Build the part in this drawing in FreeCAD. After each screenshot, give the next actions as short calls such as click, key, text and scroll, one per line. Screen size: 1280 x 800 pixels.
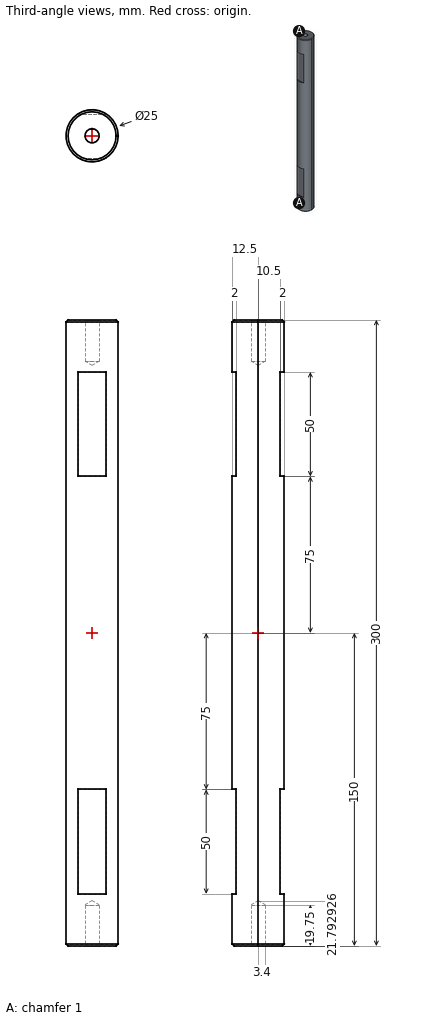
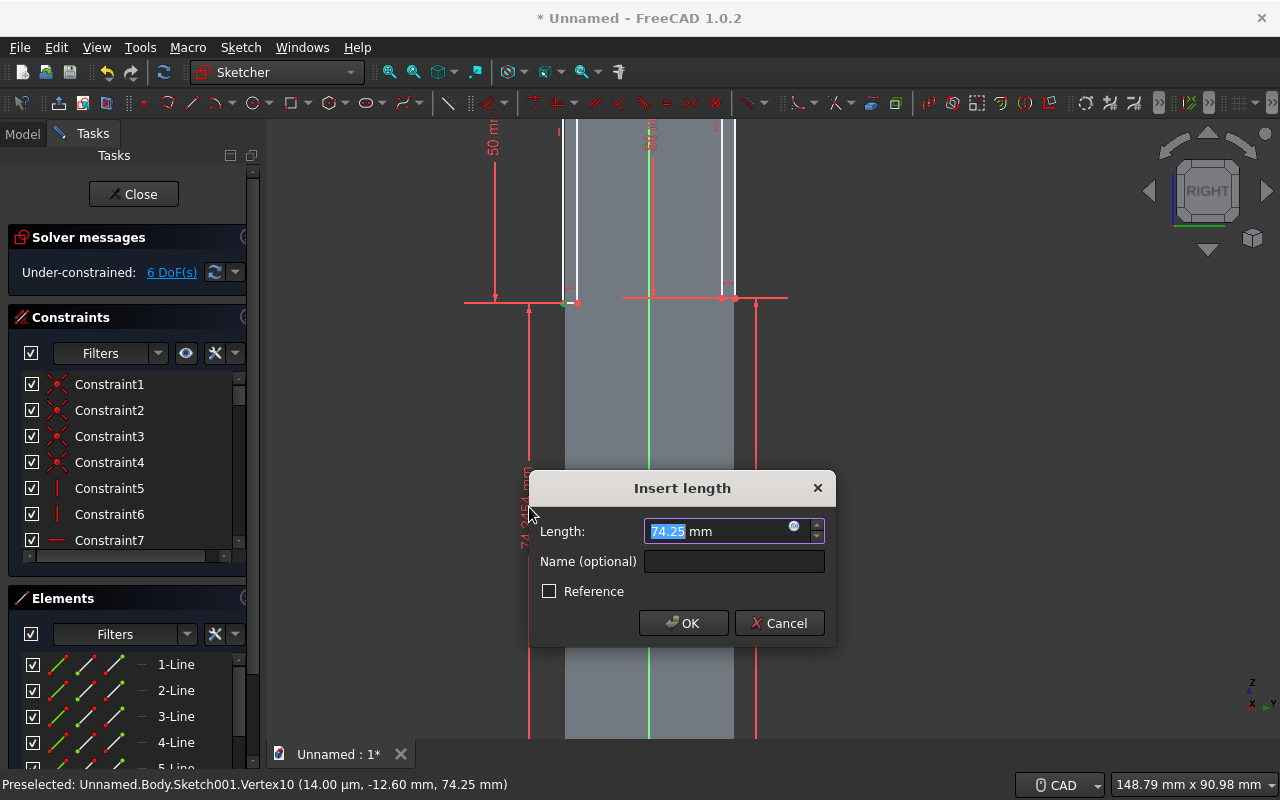
text(75)
key(Return)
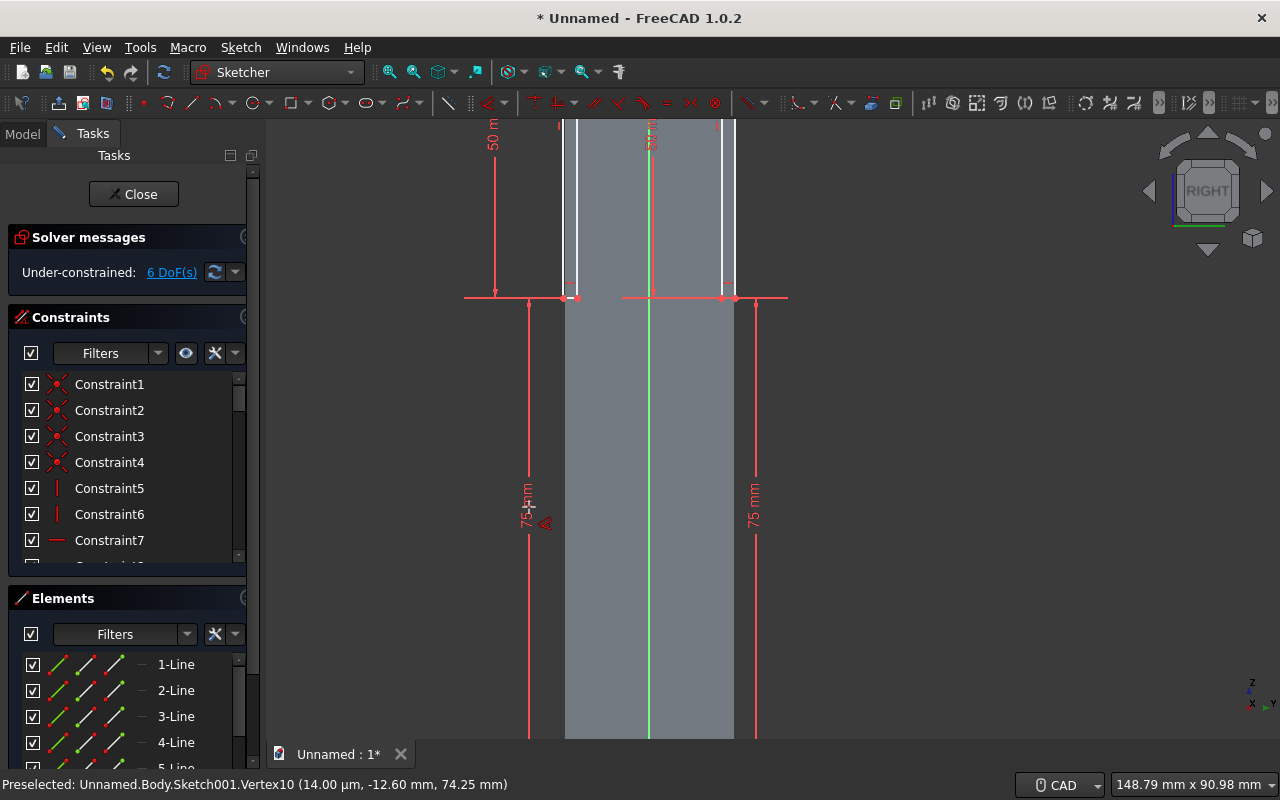
scroll(723, 305, down, 7)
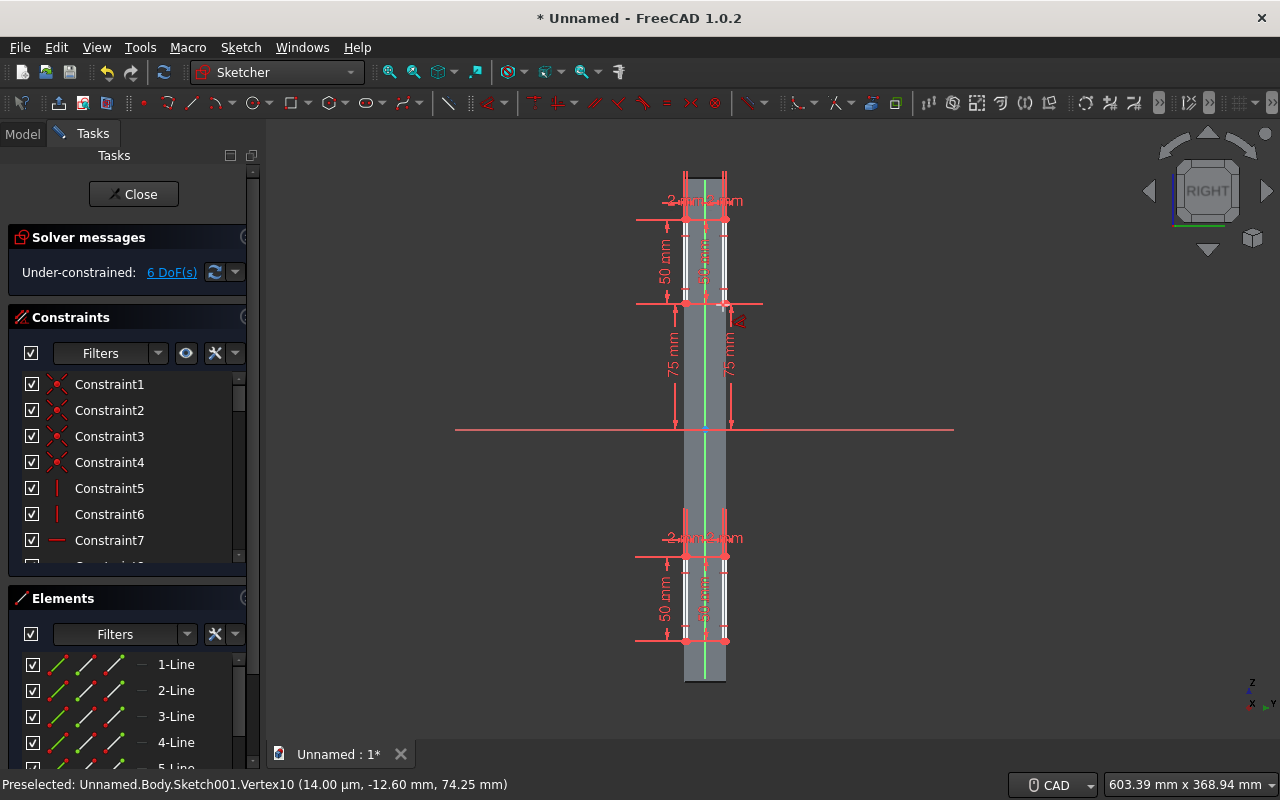
scroll(684, 557, up, 7)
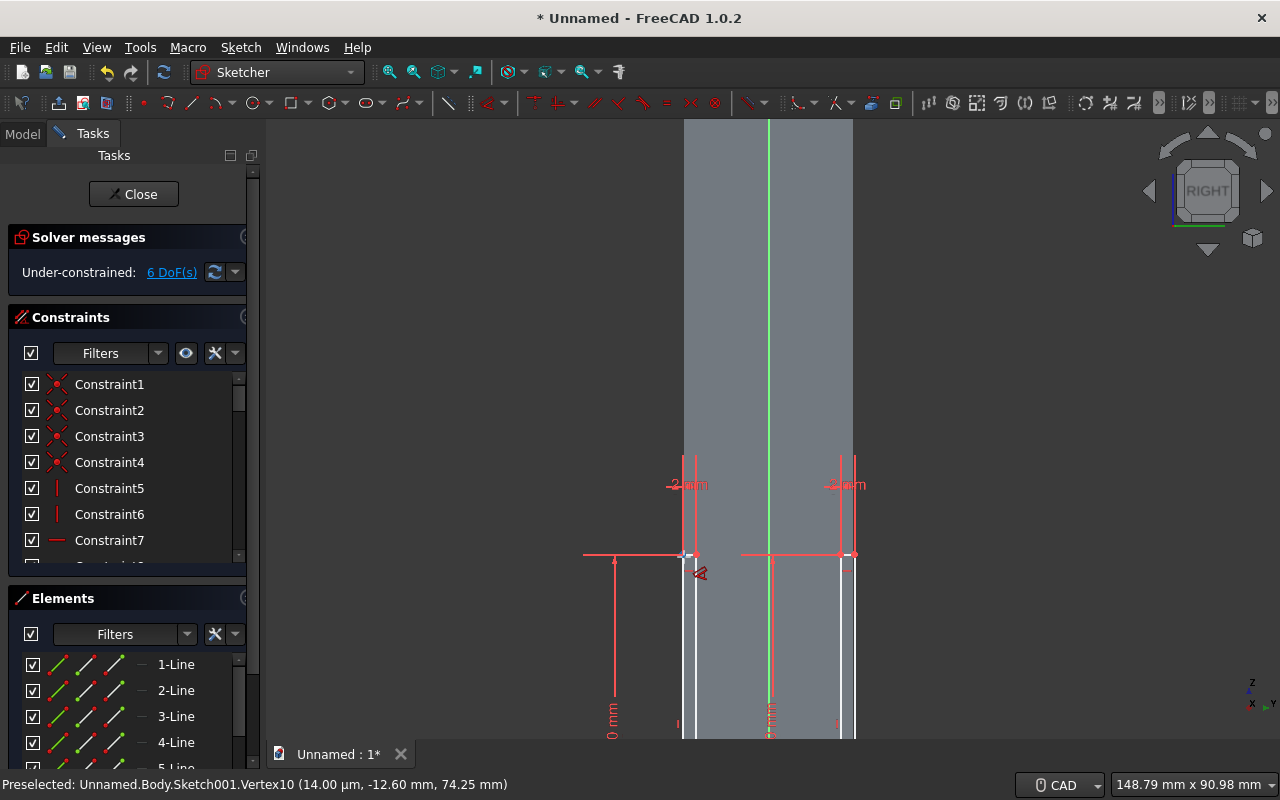
click(683, 555)
click(649, 351)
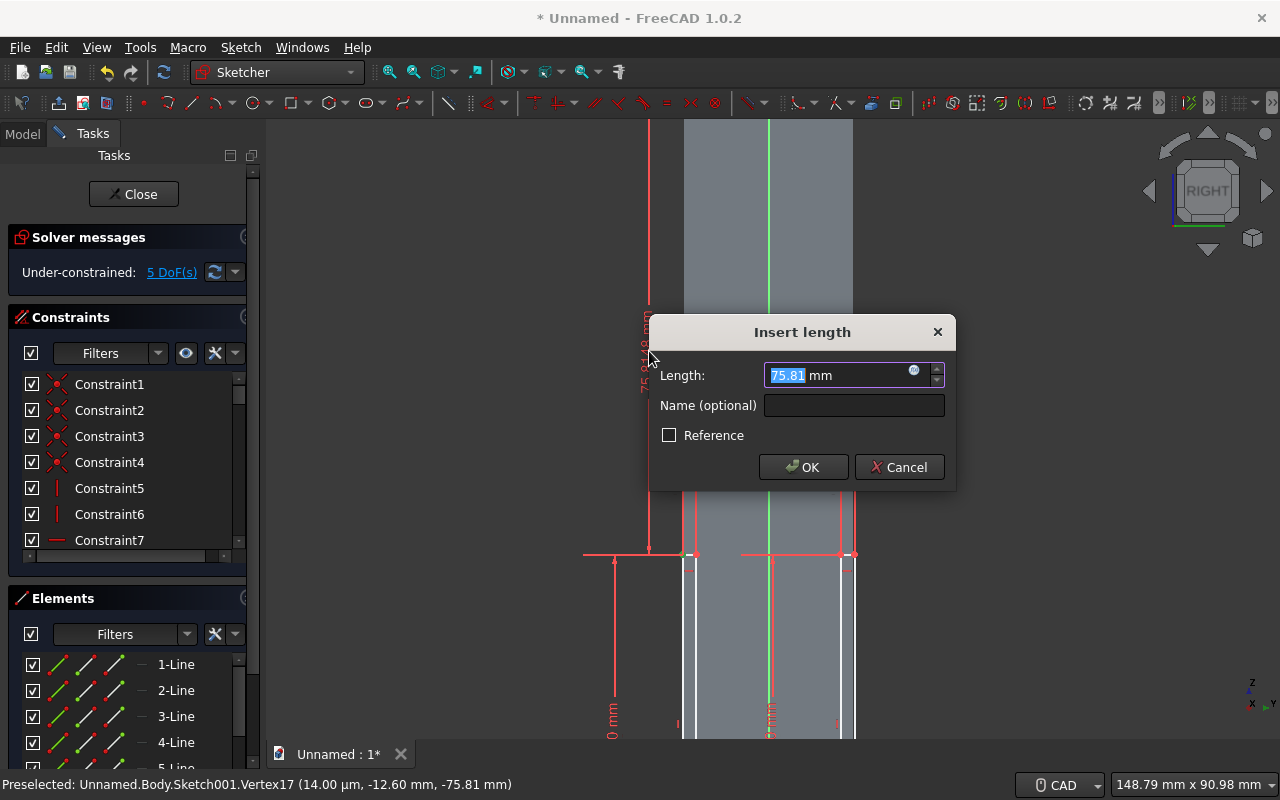
text(75)
key(Return)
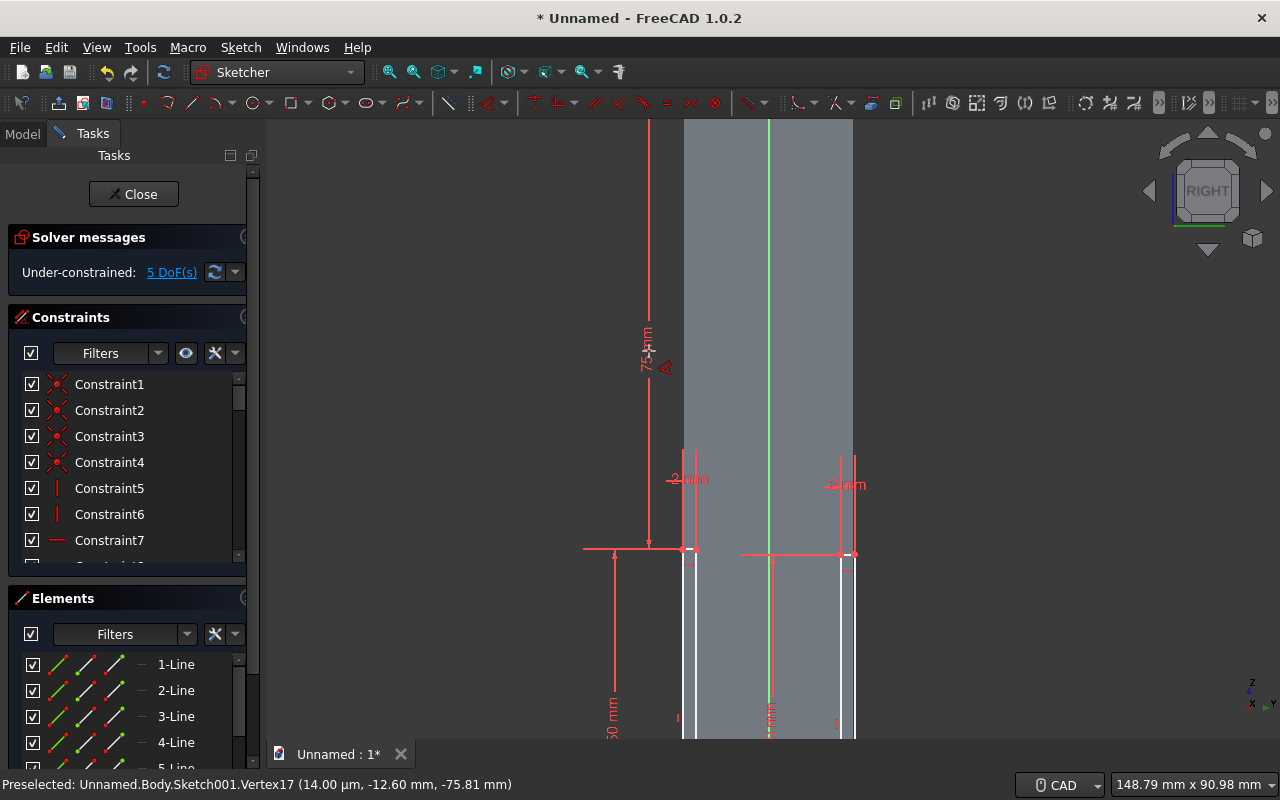
click(841, 555)
click(875, 351)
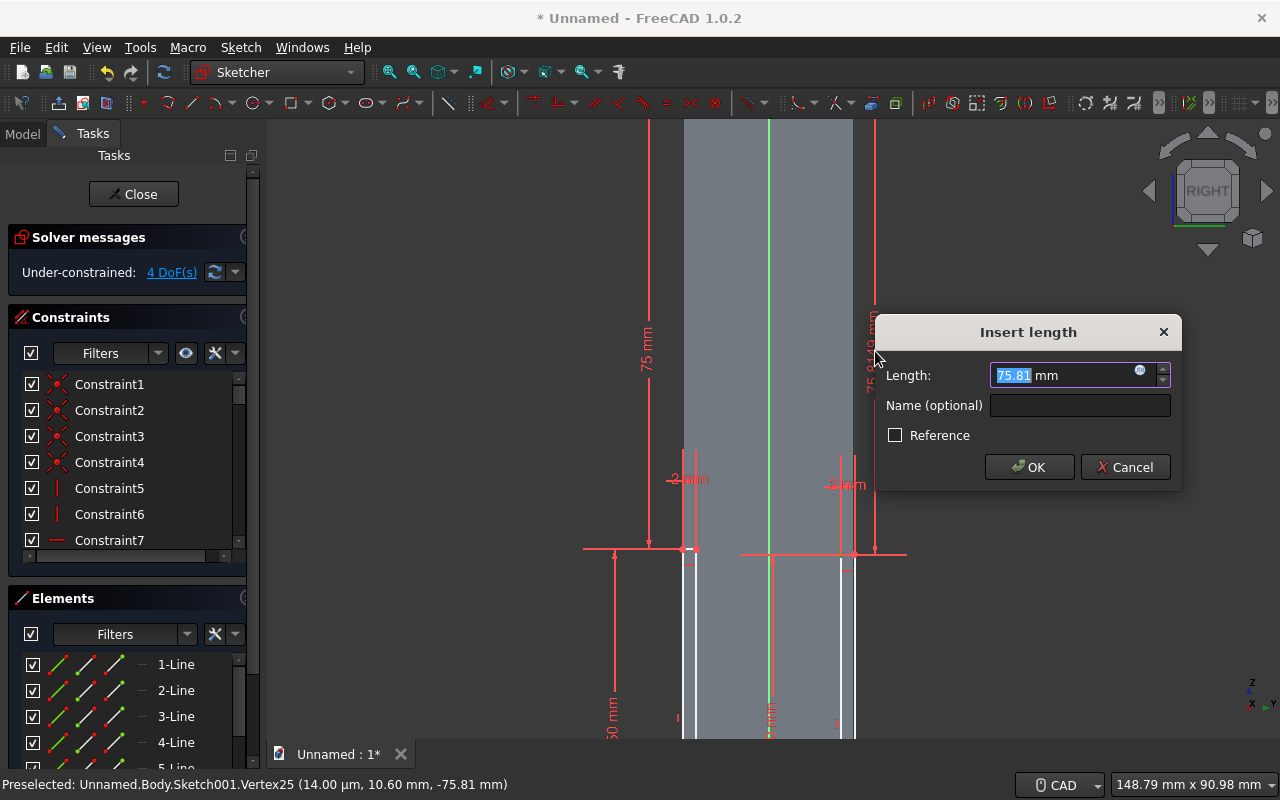
text(75)
key(Return)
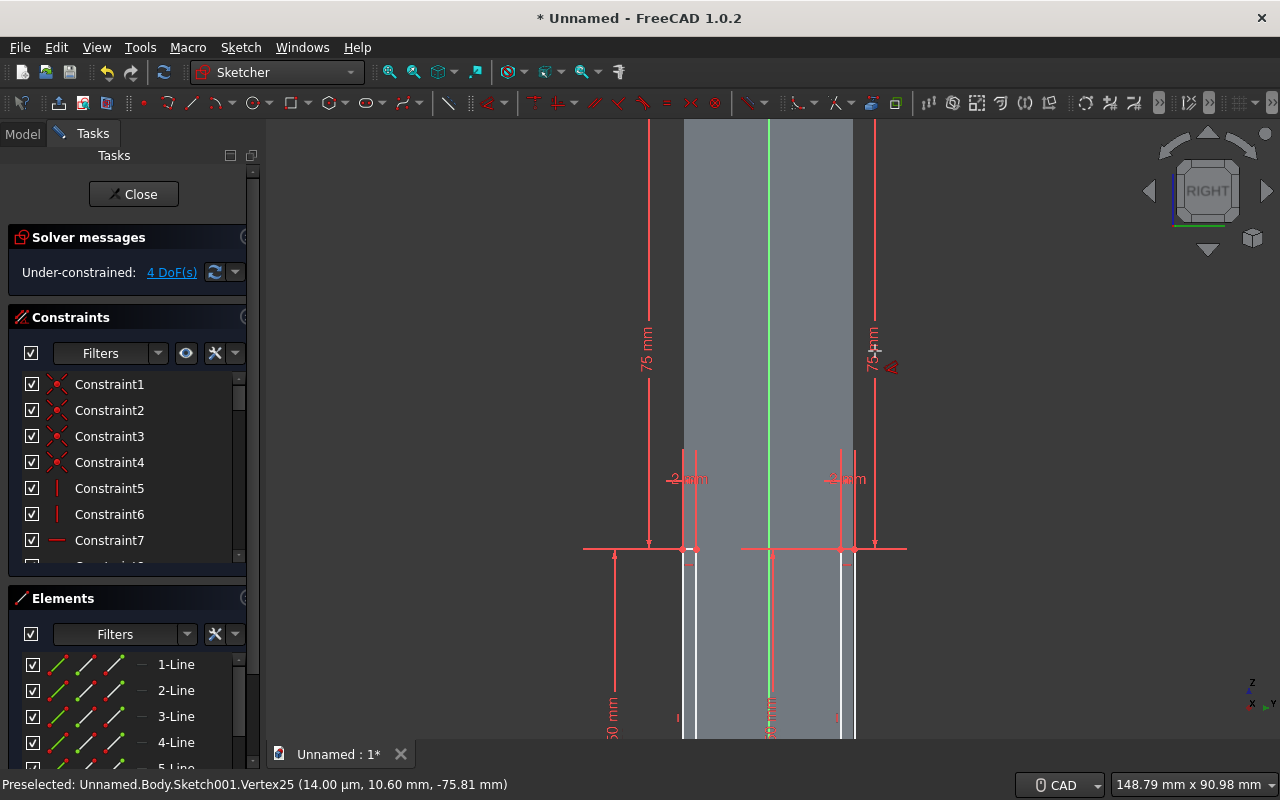
scroll(684, 557, down, 7)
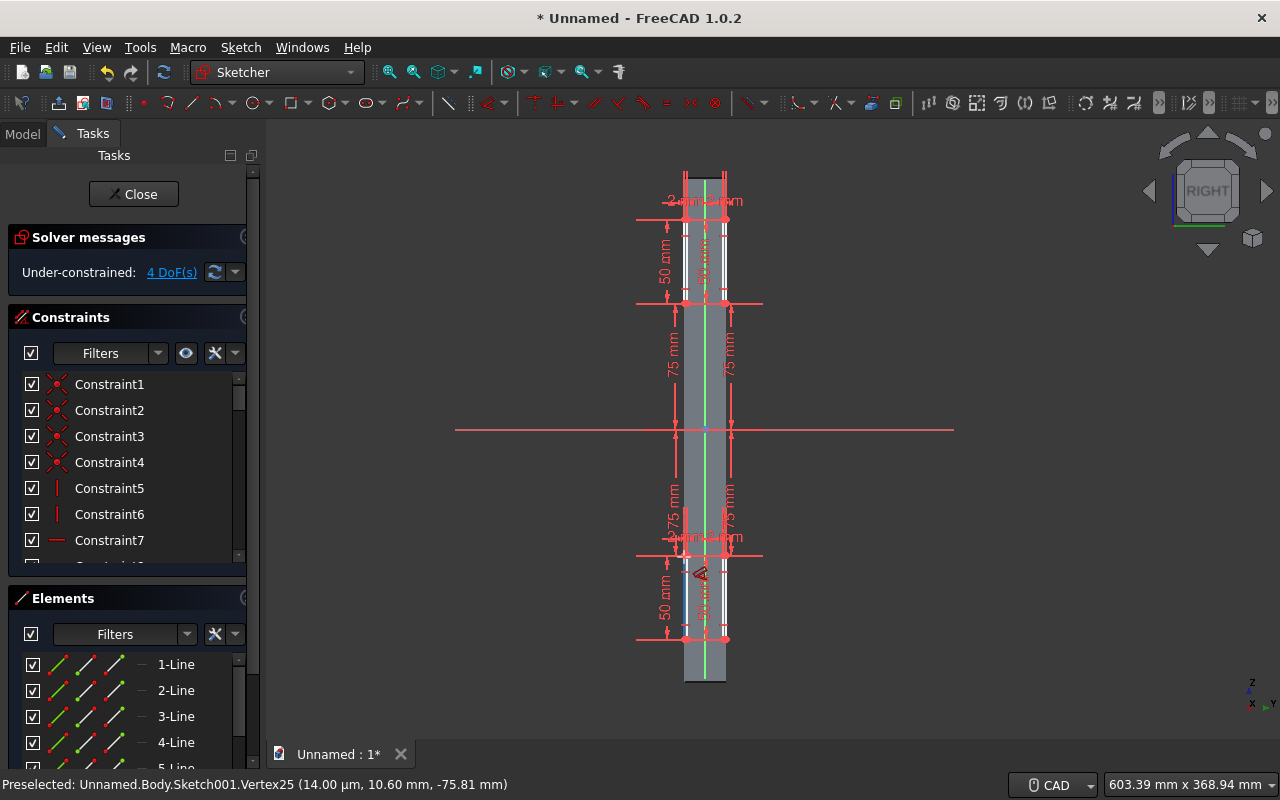
scroll(723, 220, up, 7)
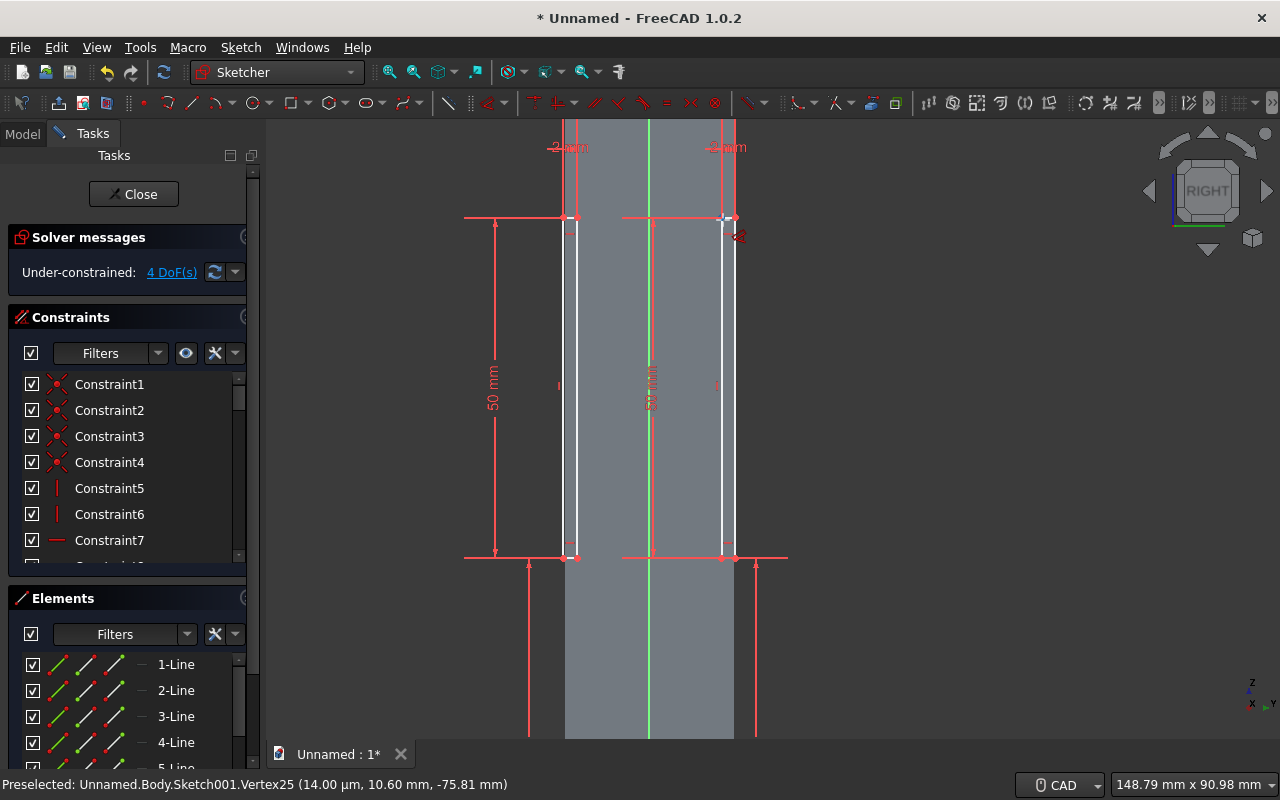
click(722, 218)
click(685, 184)